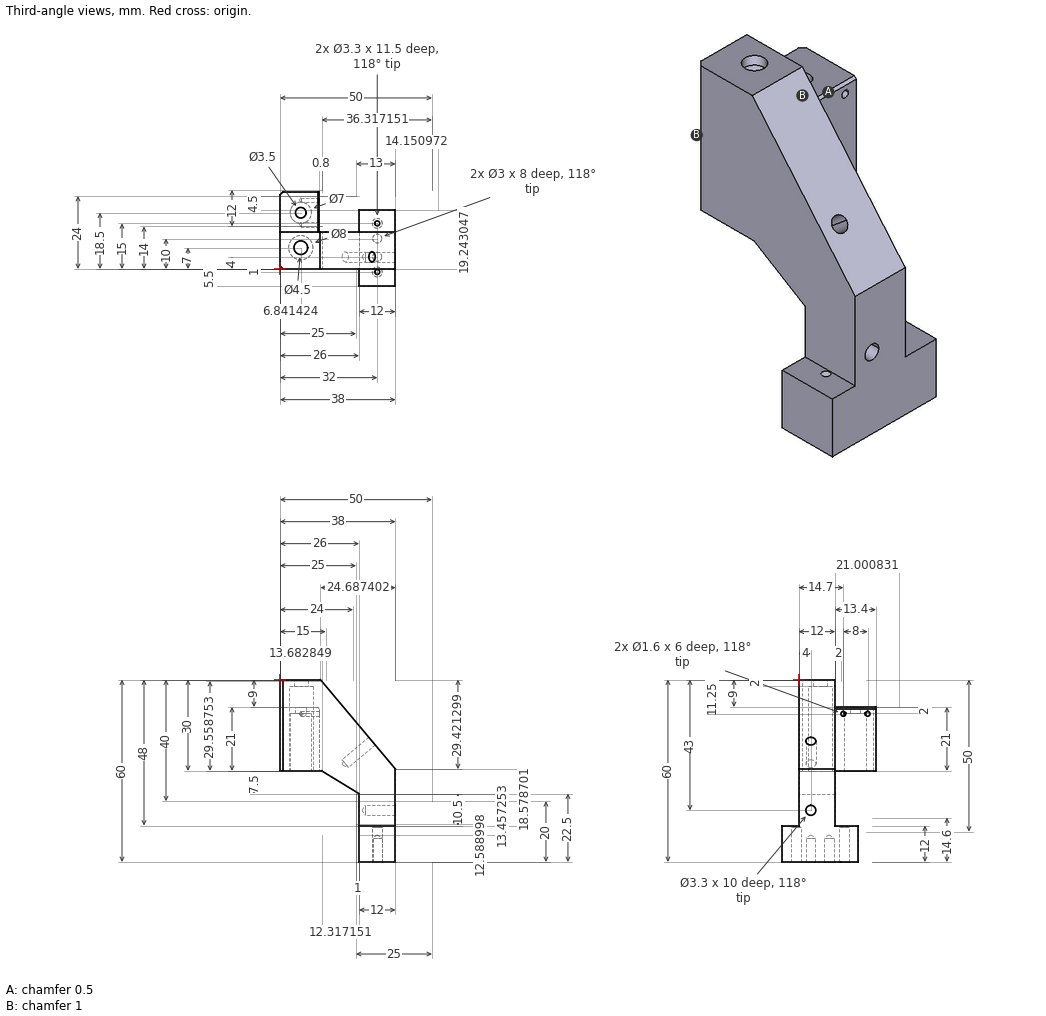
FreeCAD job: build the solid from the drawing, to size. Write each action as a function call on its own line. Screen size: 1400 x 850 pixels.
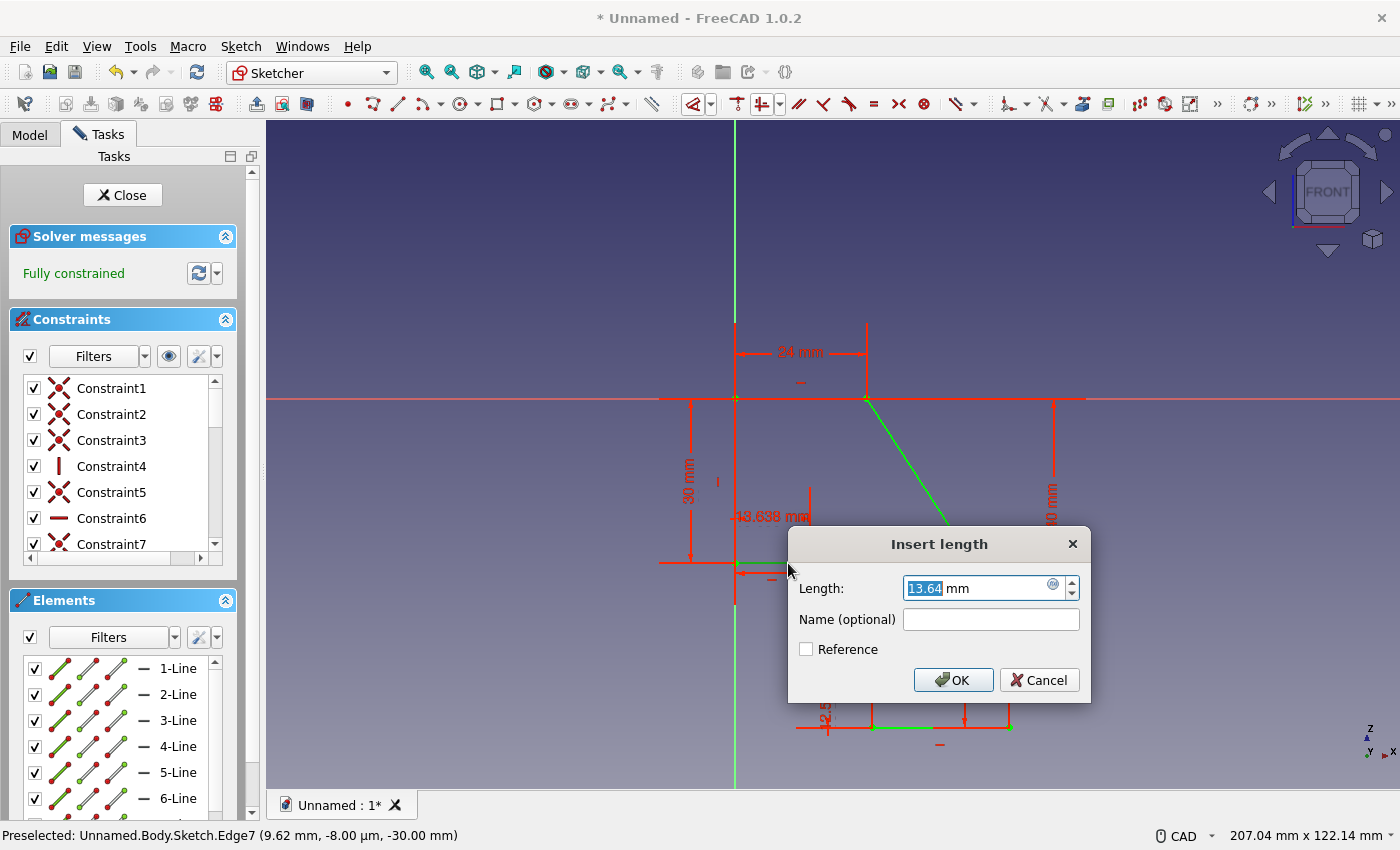
text(13.682849)
key(Return)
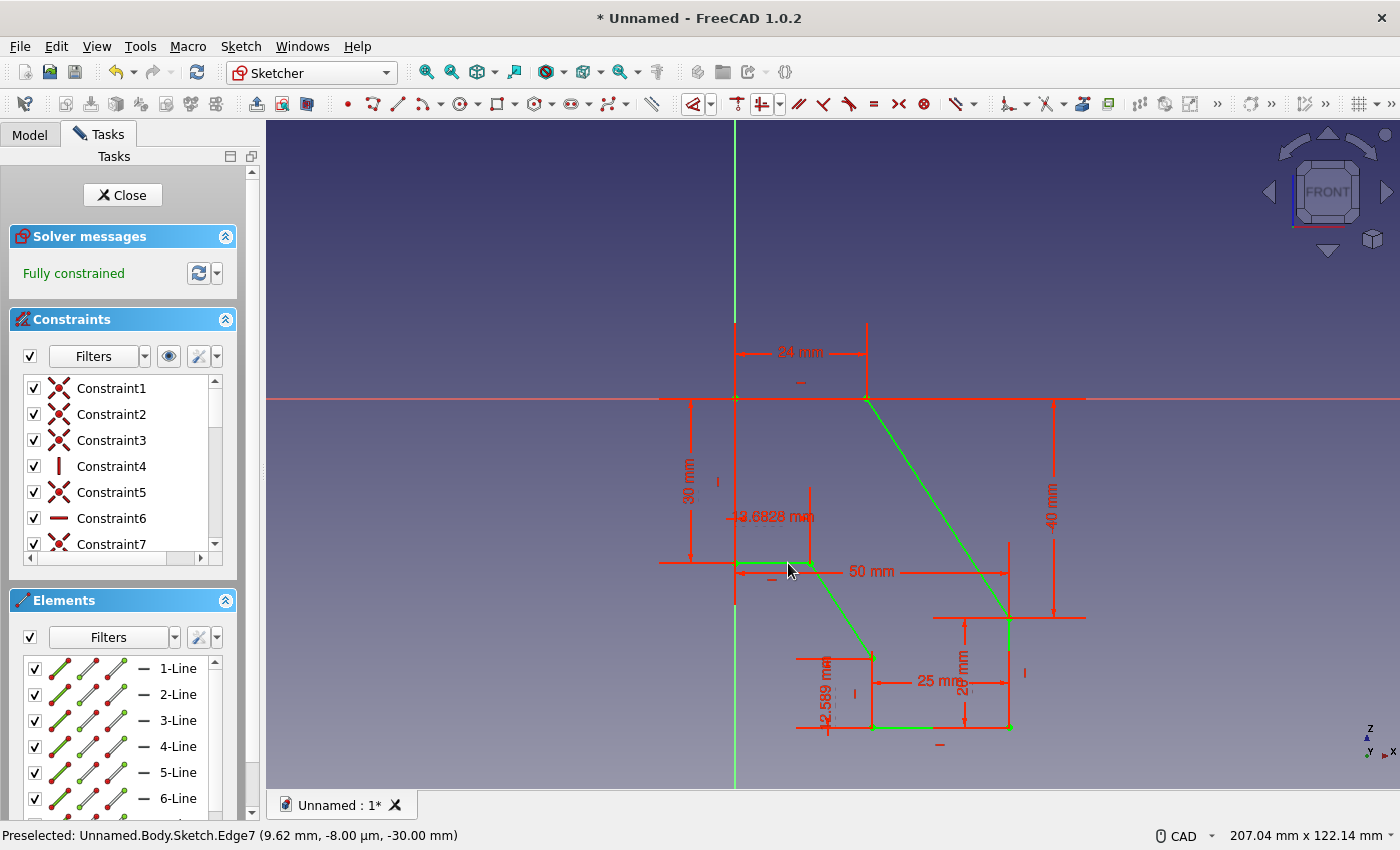
click(123, 195)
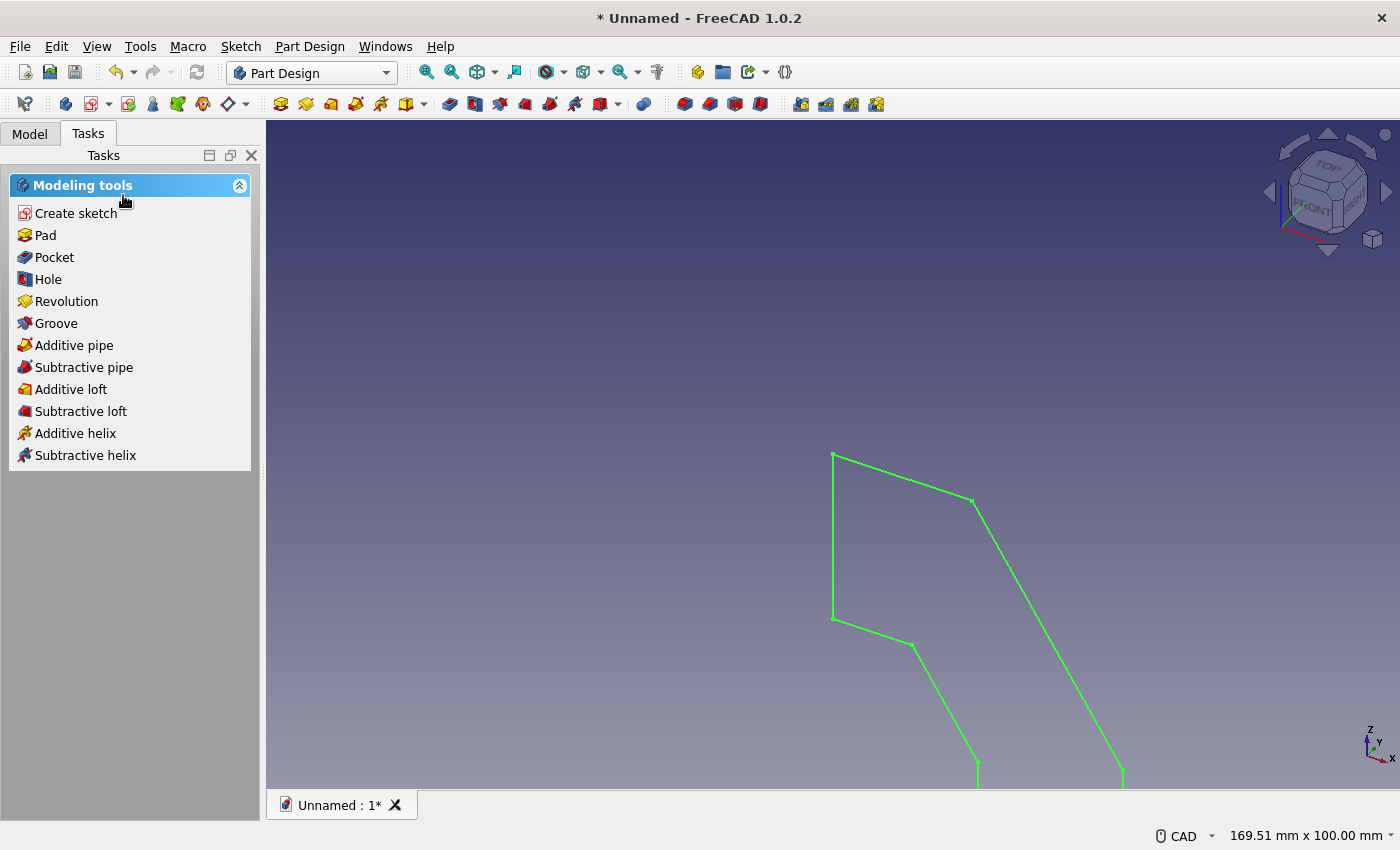
click(281, 104)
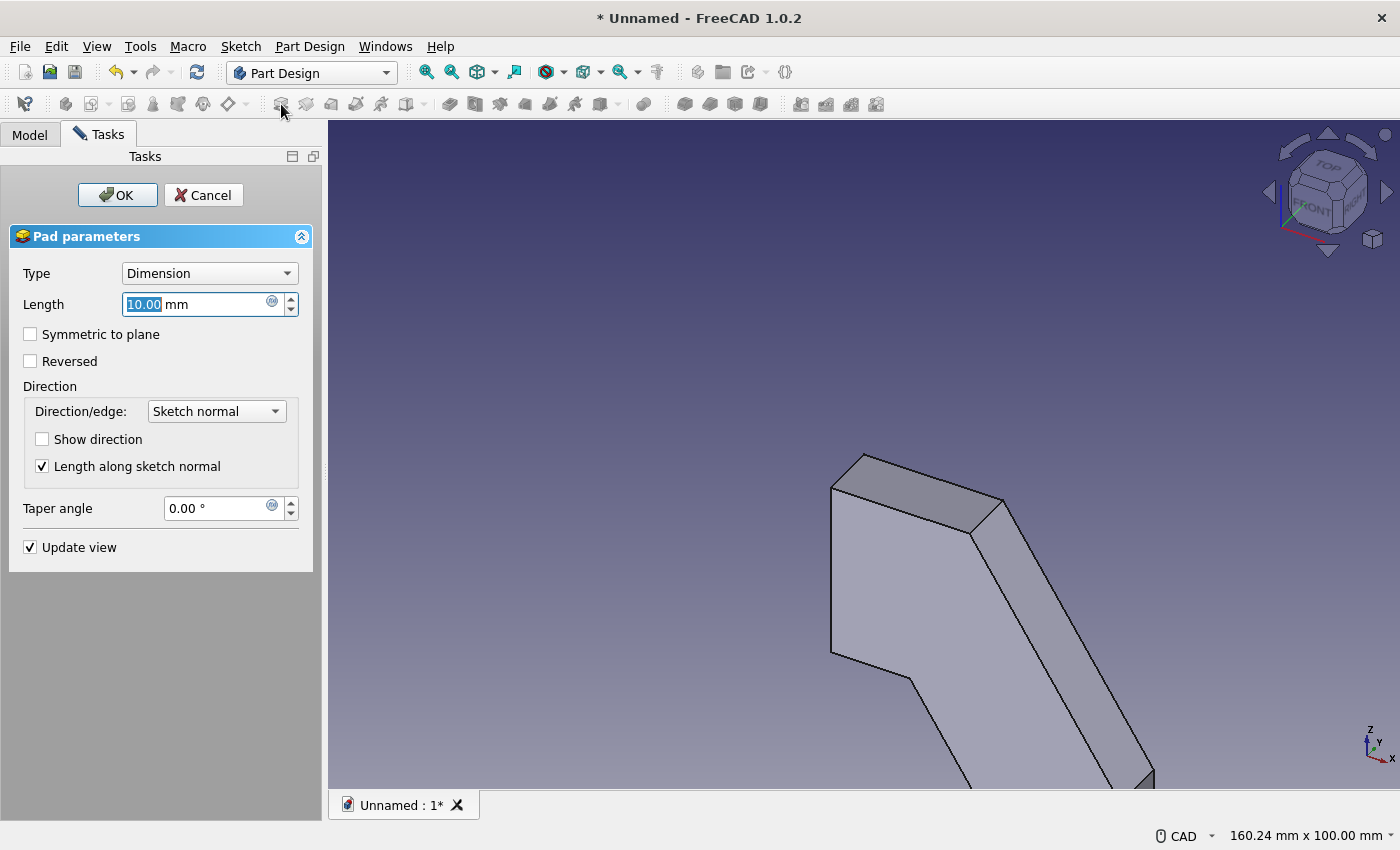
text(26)
key(Tab)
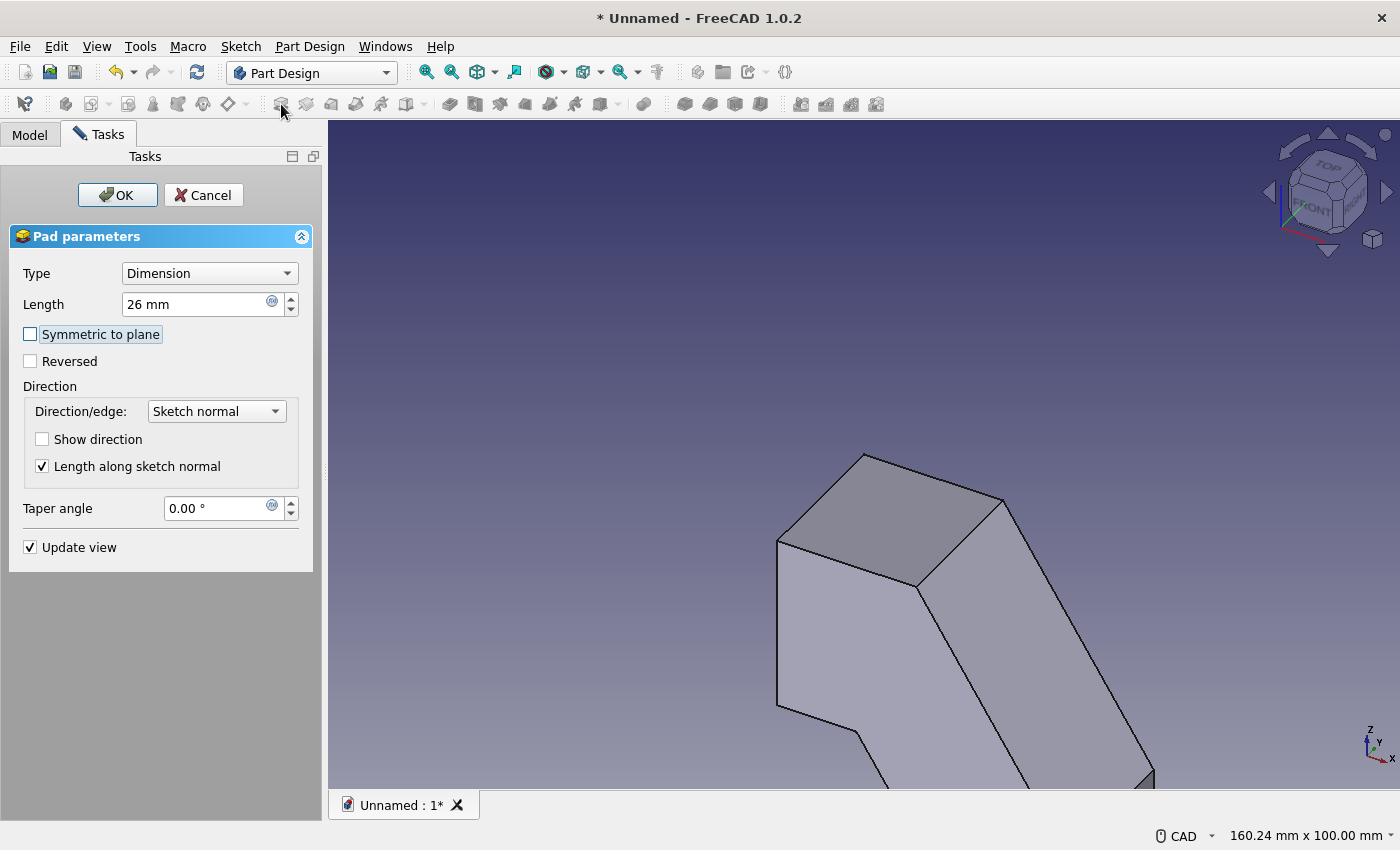
click(31, 361)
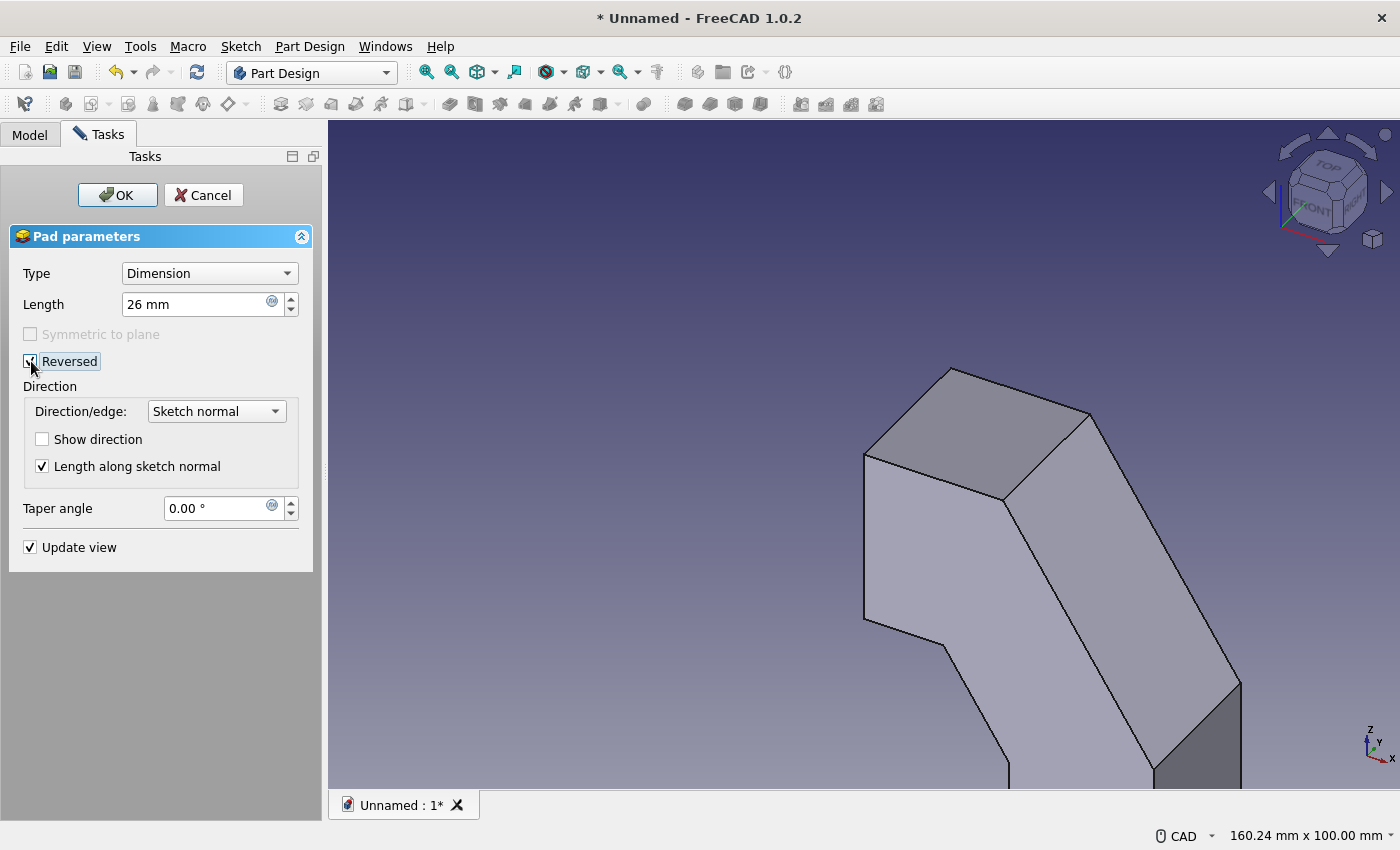
click(118, 195)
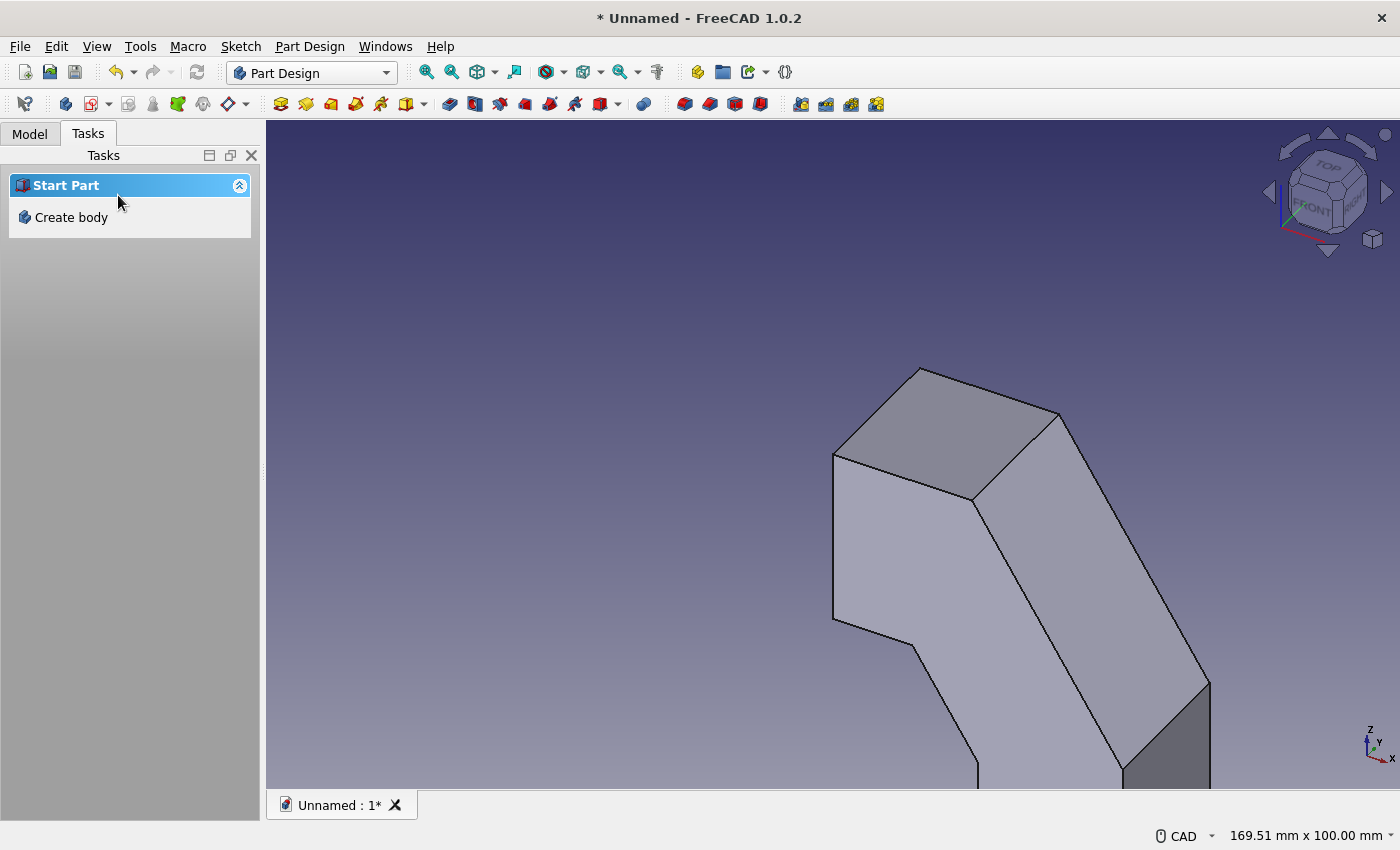
click(427, 72)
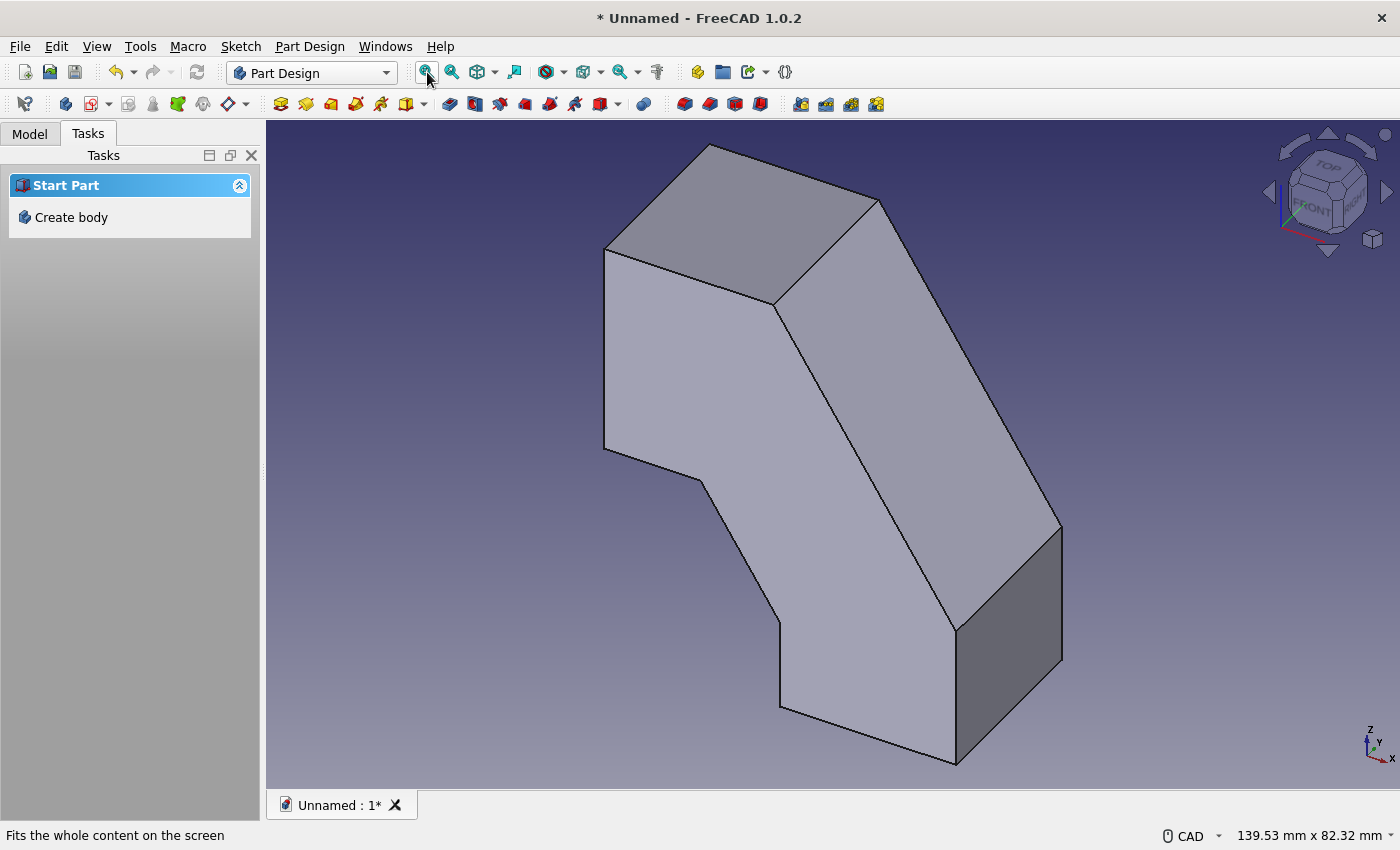
key(5)